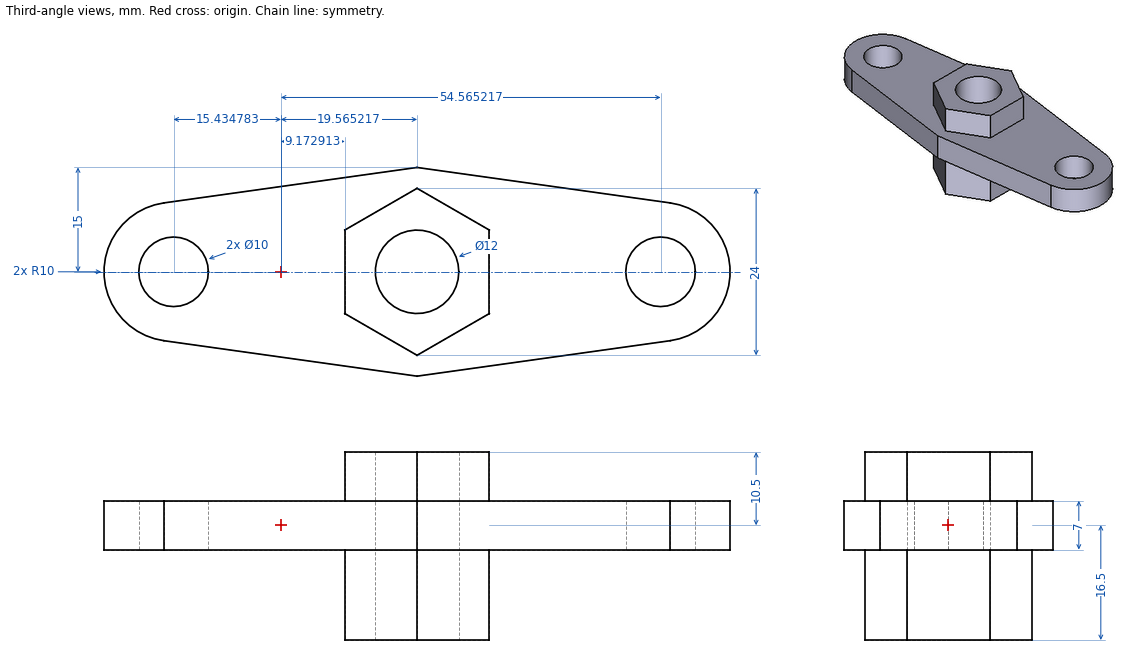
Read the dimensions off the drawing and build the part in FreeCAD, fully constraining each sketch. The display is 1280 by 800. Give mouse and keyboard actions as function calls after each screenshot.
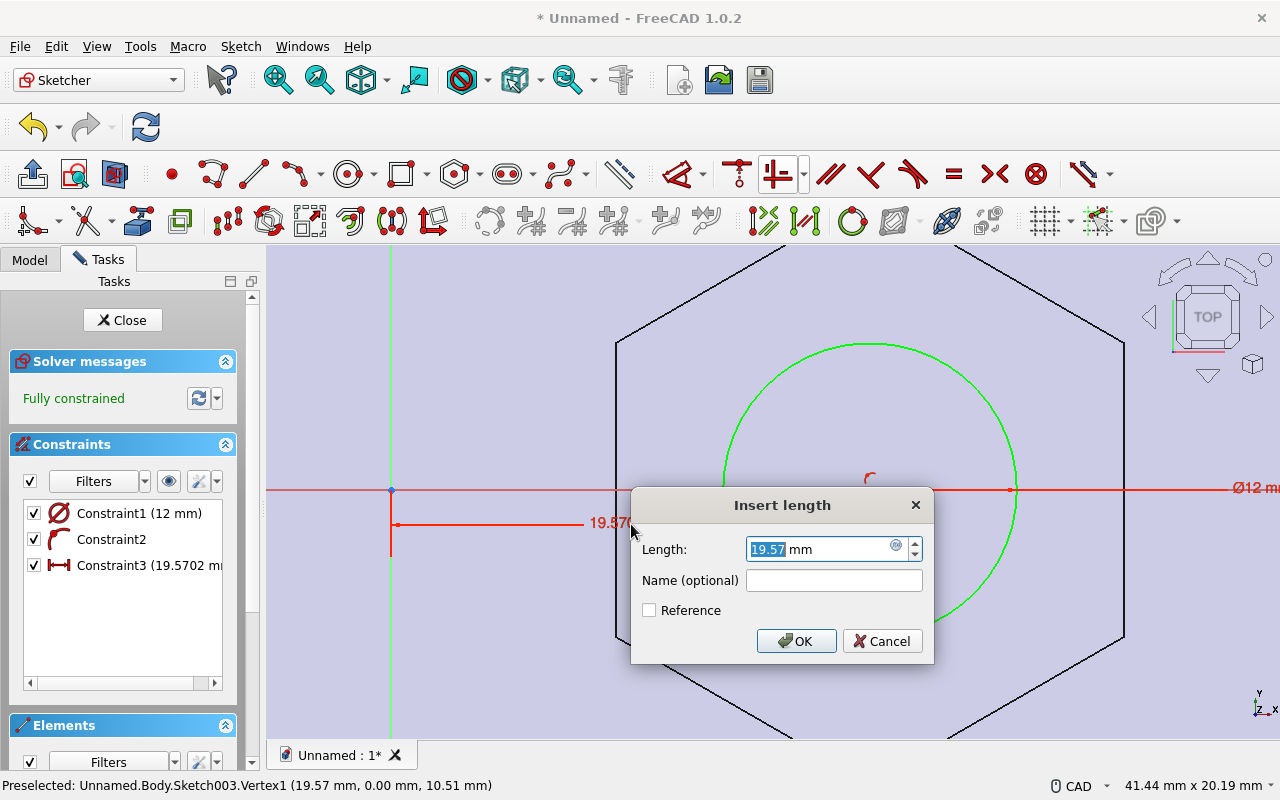
text(19.565217)
key(Return)
key(Escape)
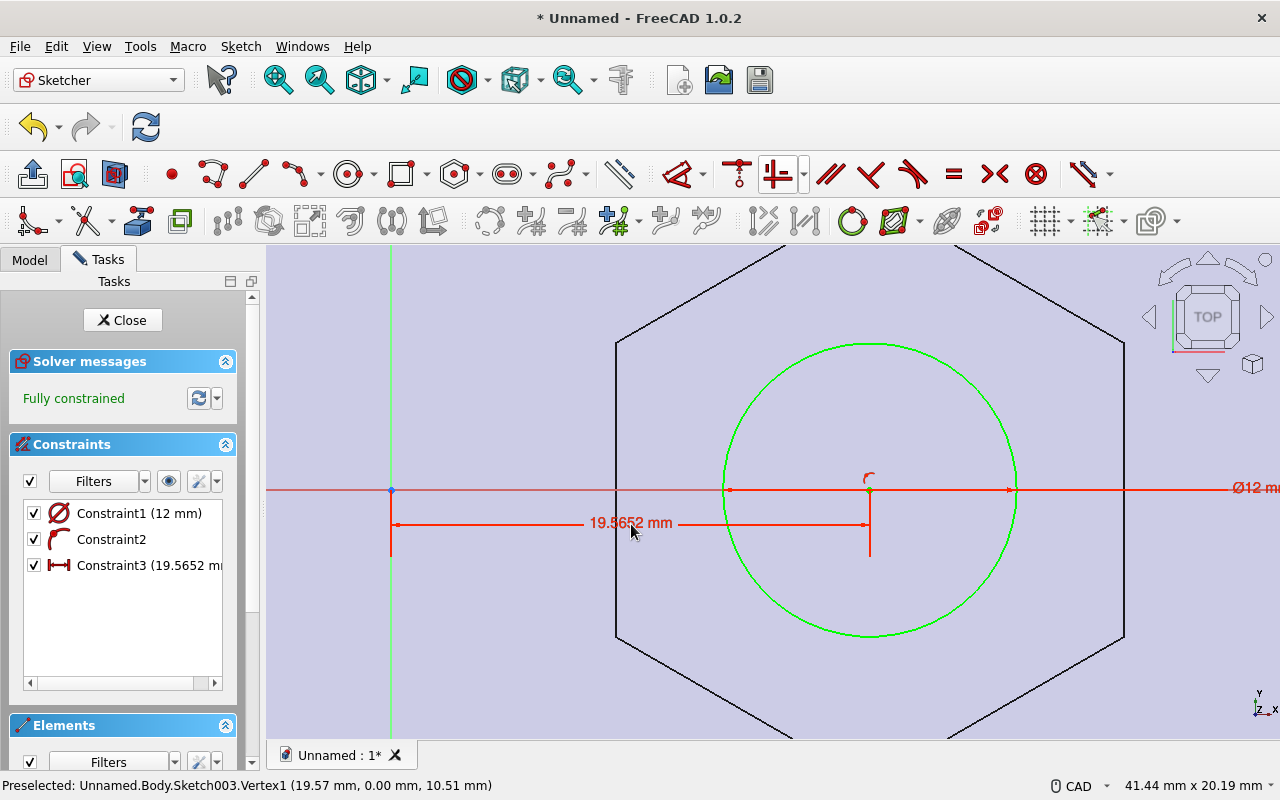
click(123, 320)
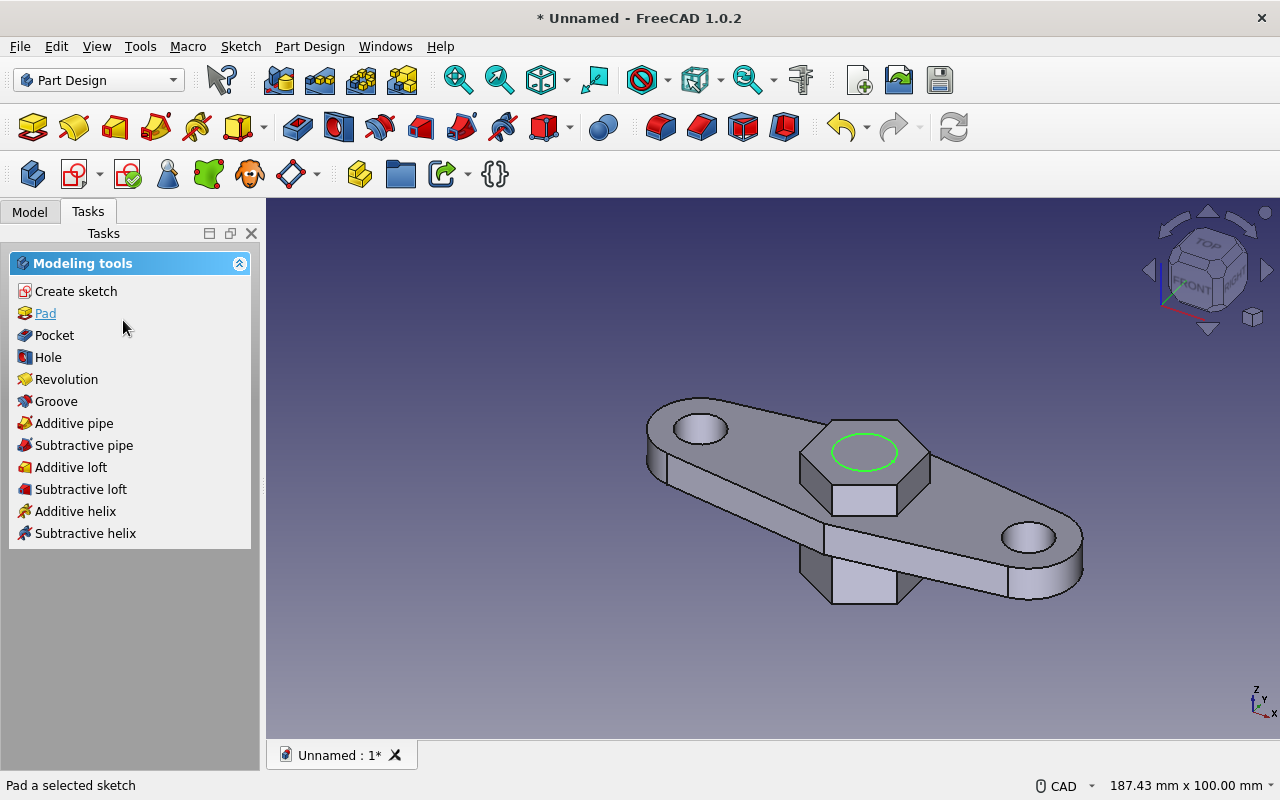
click(298, 128)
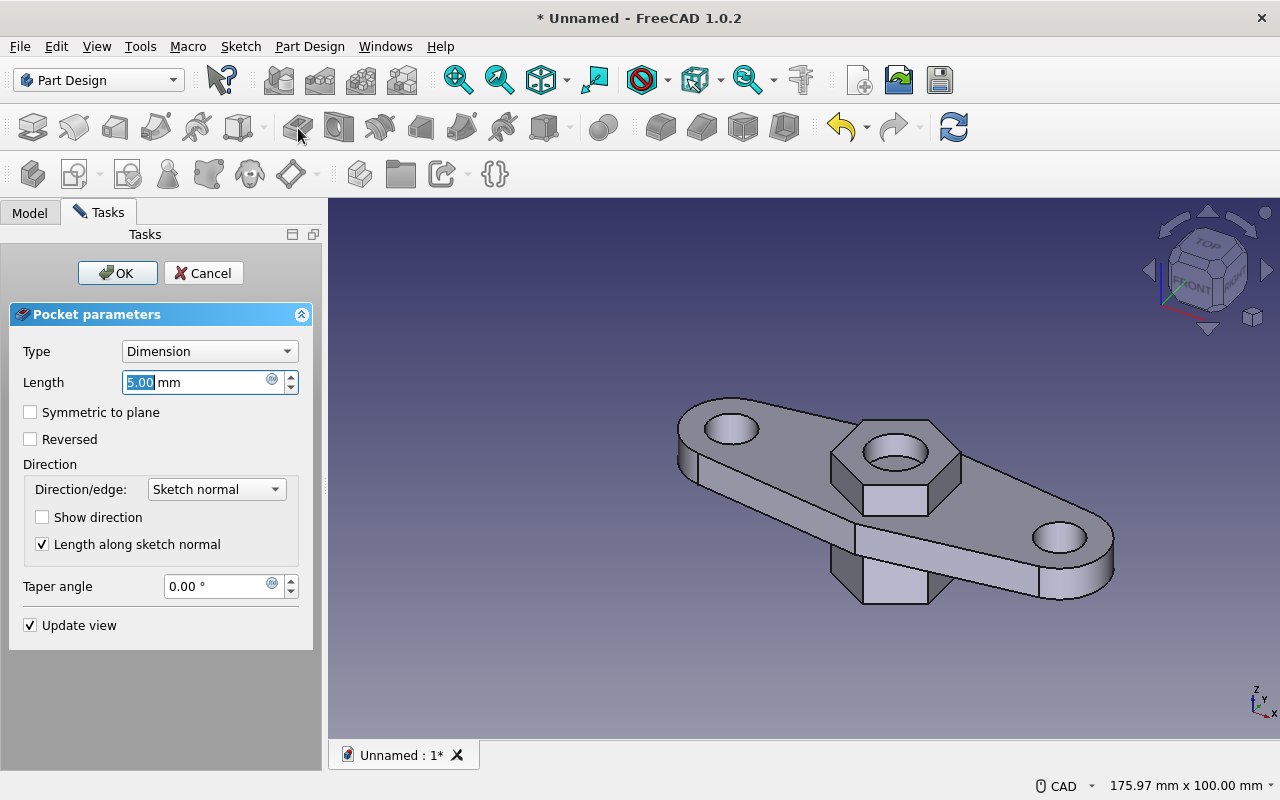
click(210, 352)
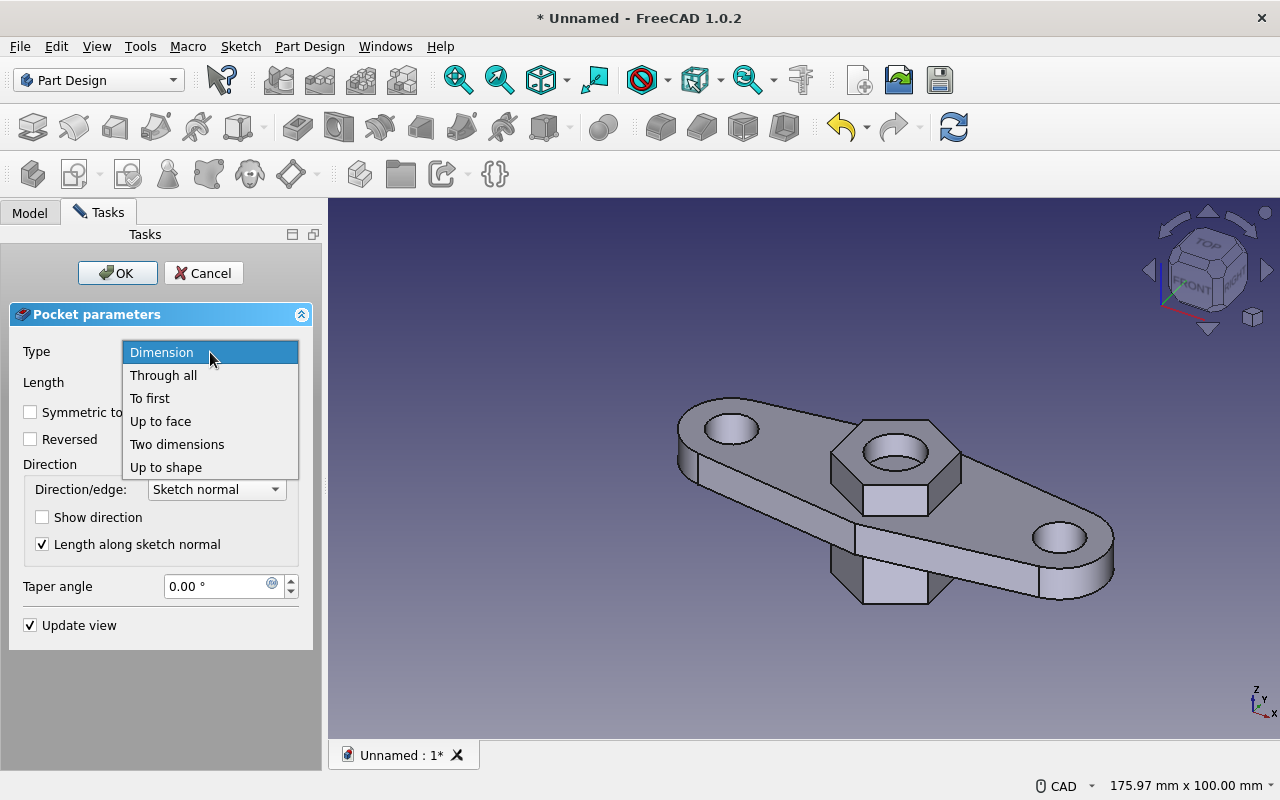
click(208, 376)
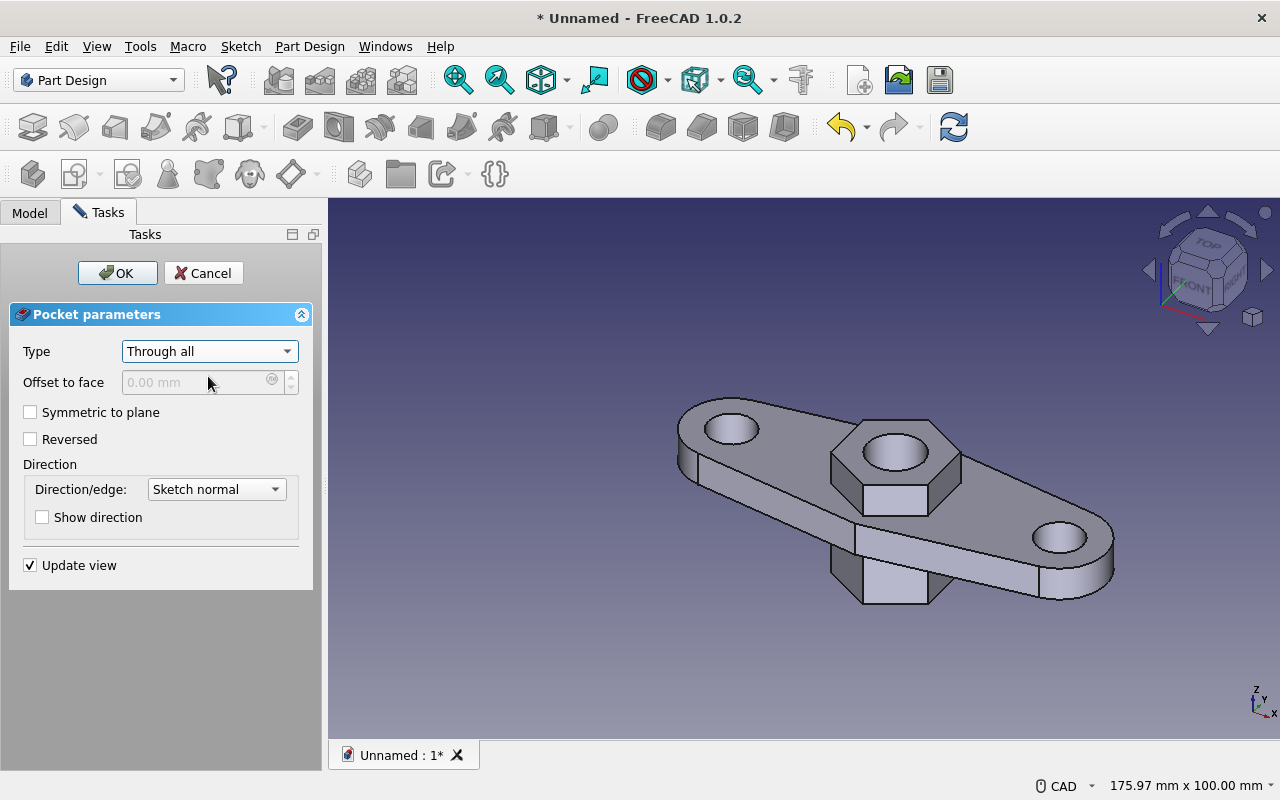
click(118, 273)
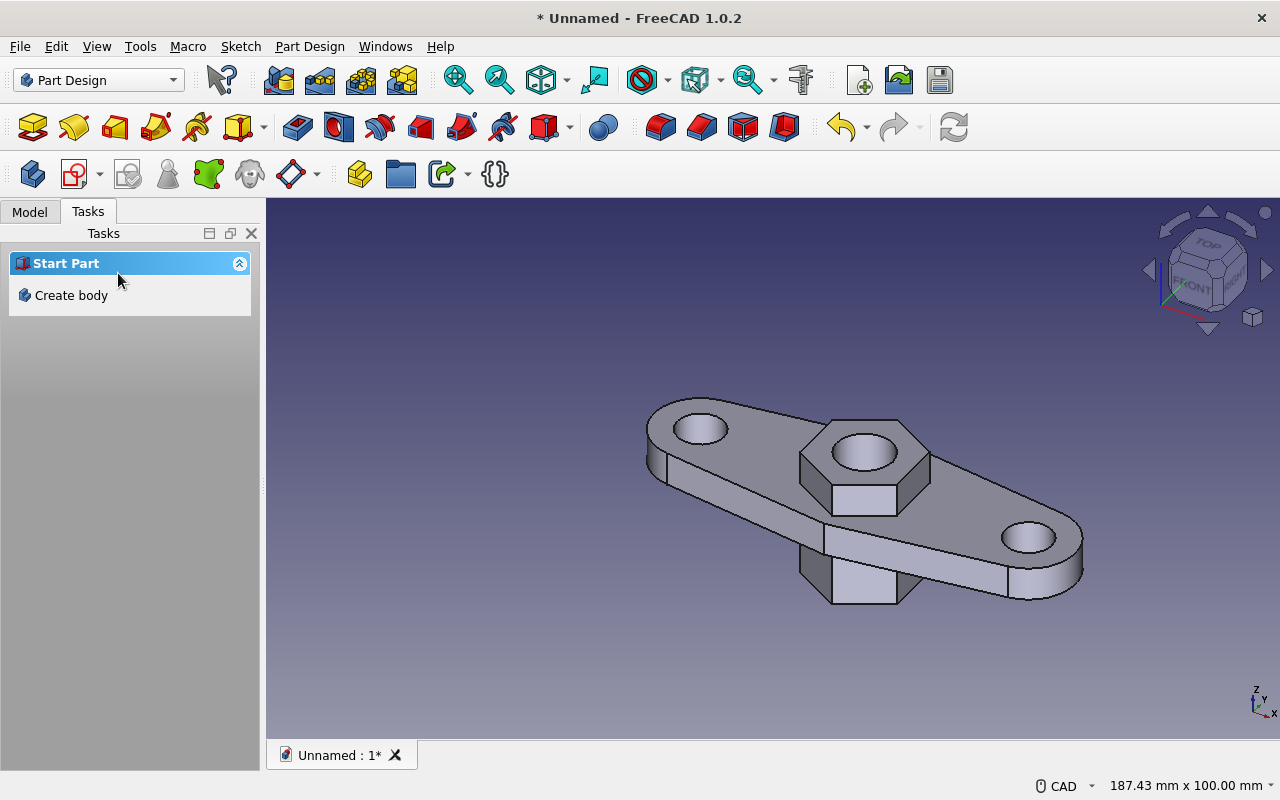
key(0)